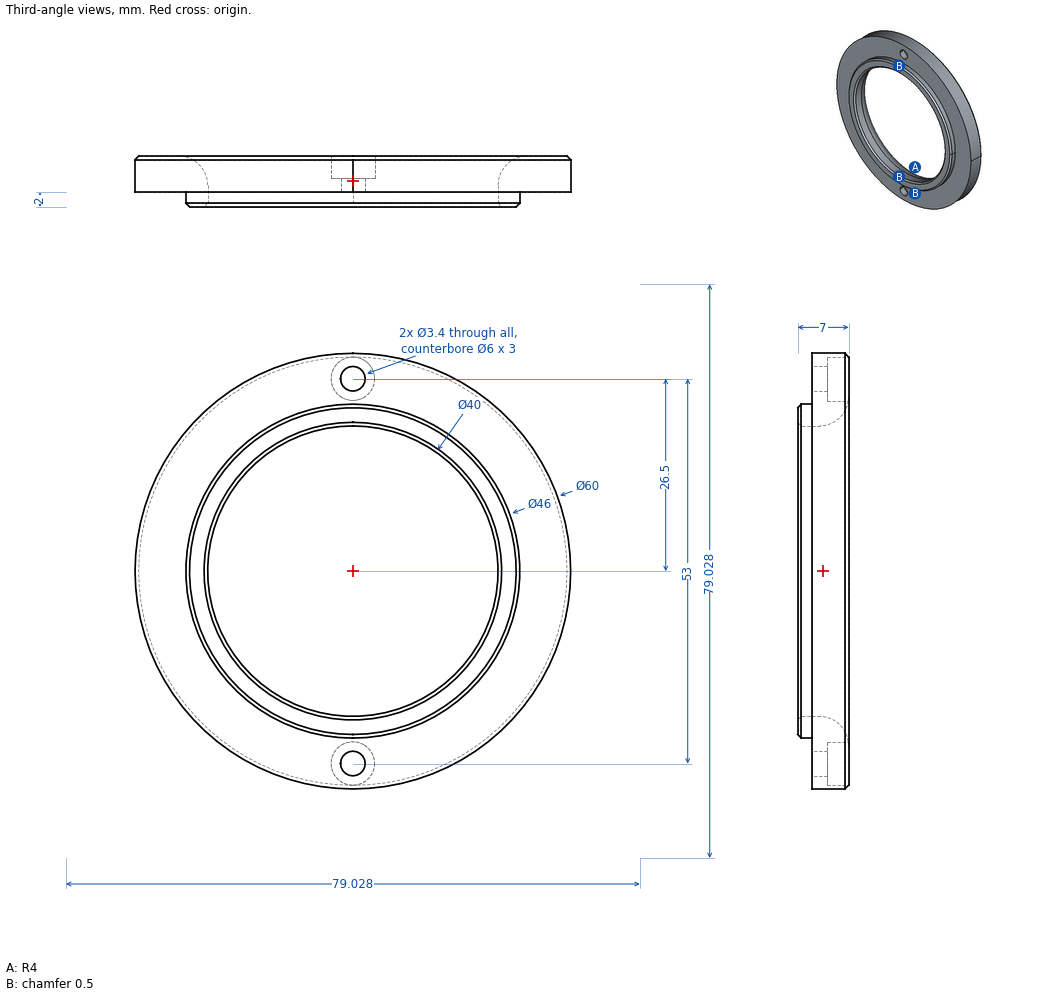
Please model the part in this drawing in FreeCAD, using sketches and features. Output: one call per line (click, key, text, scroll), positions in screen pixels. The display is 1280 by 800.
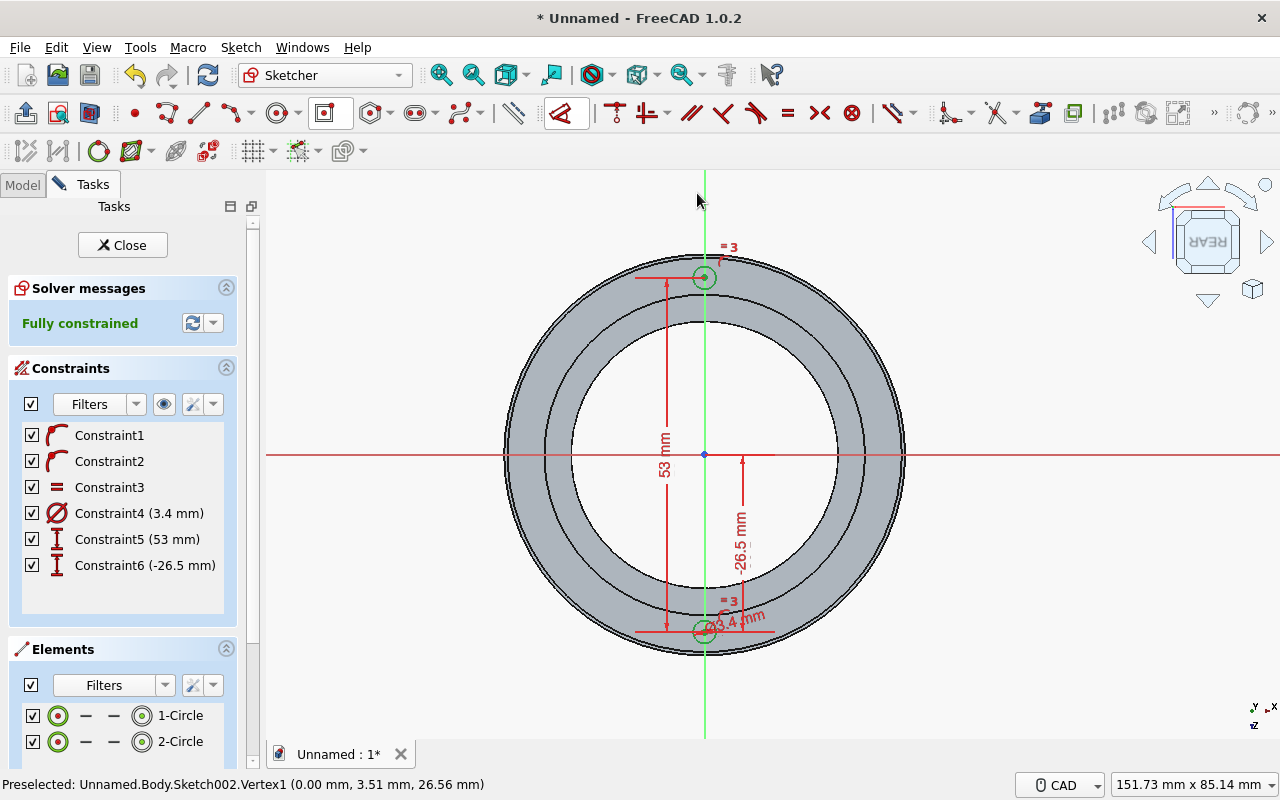
click(123, 245)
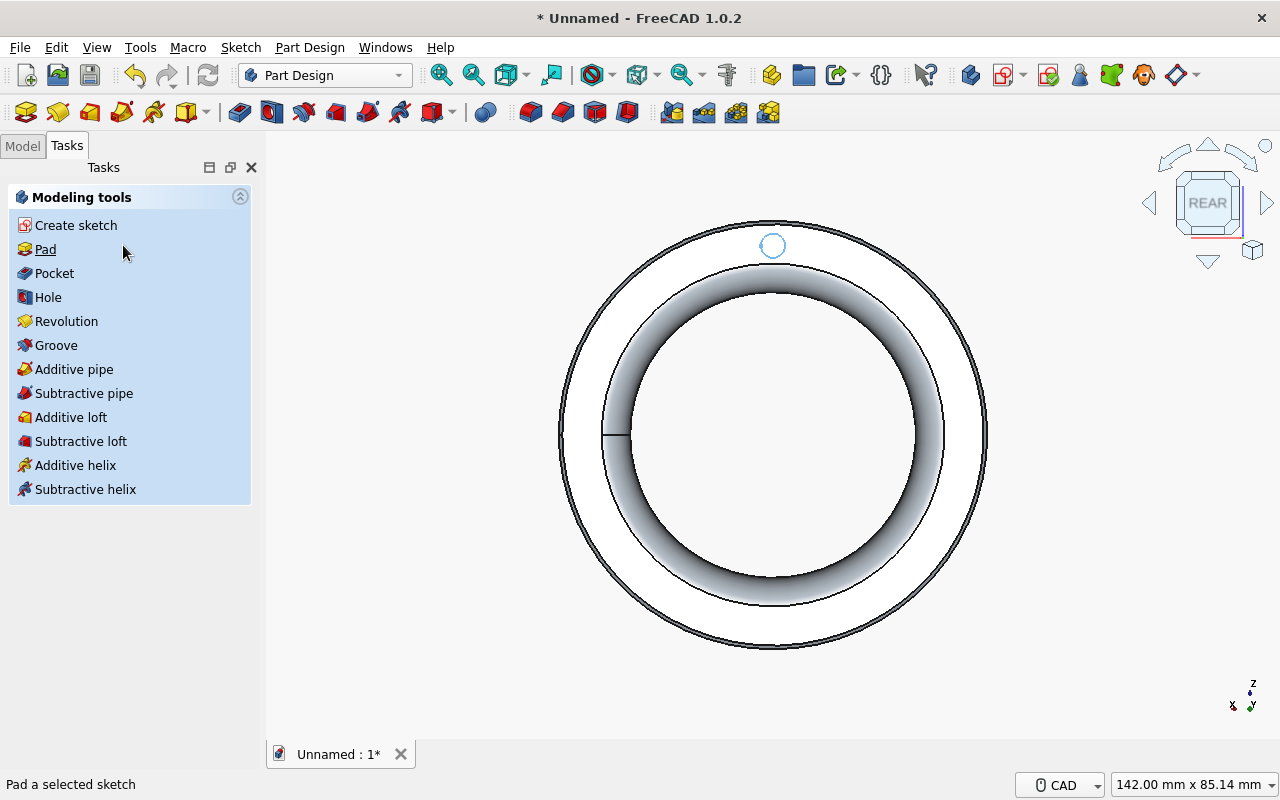
click(272, 112)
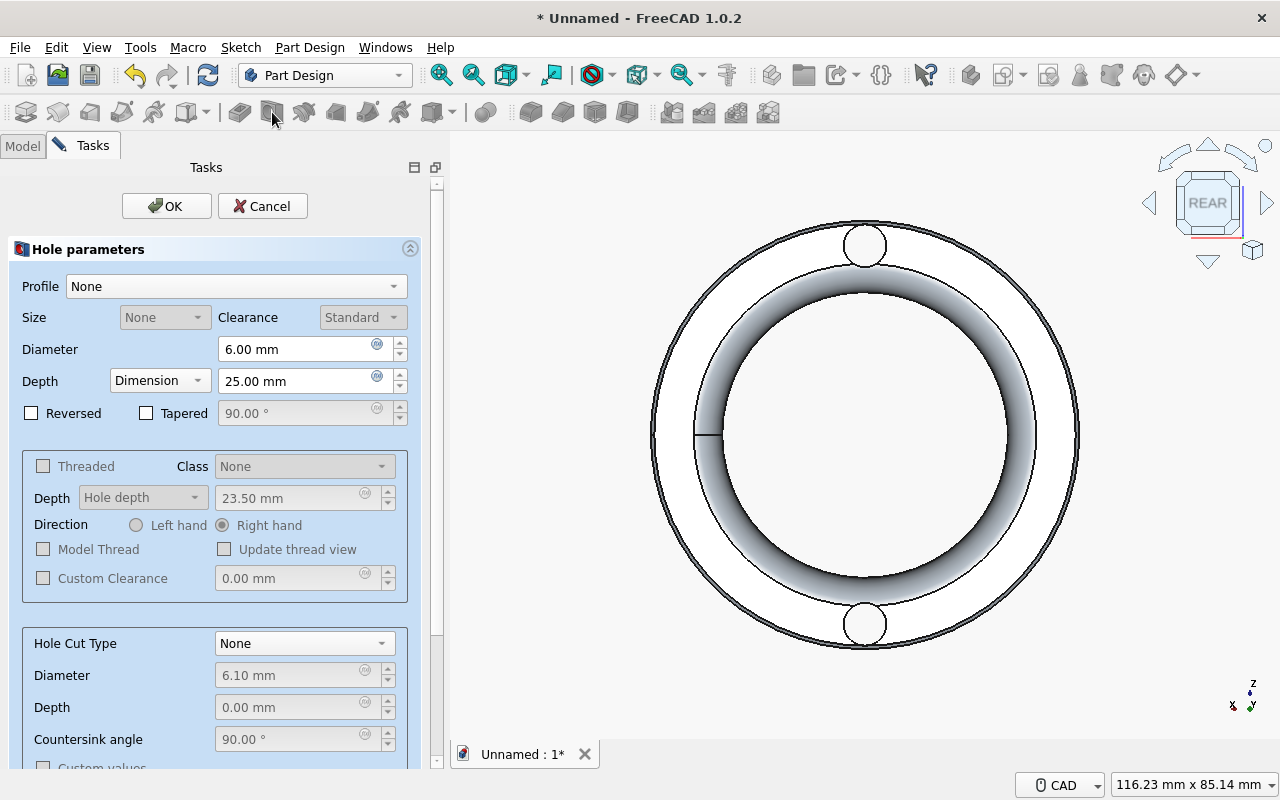
triple_click(305, 349)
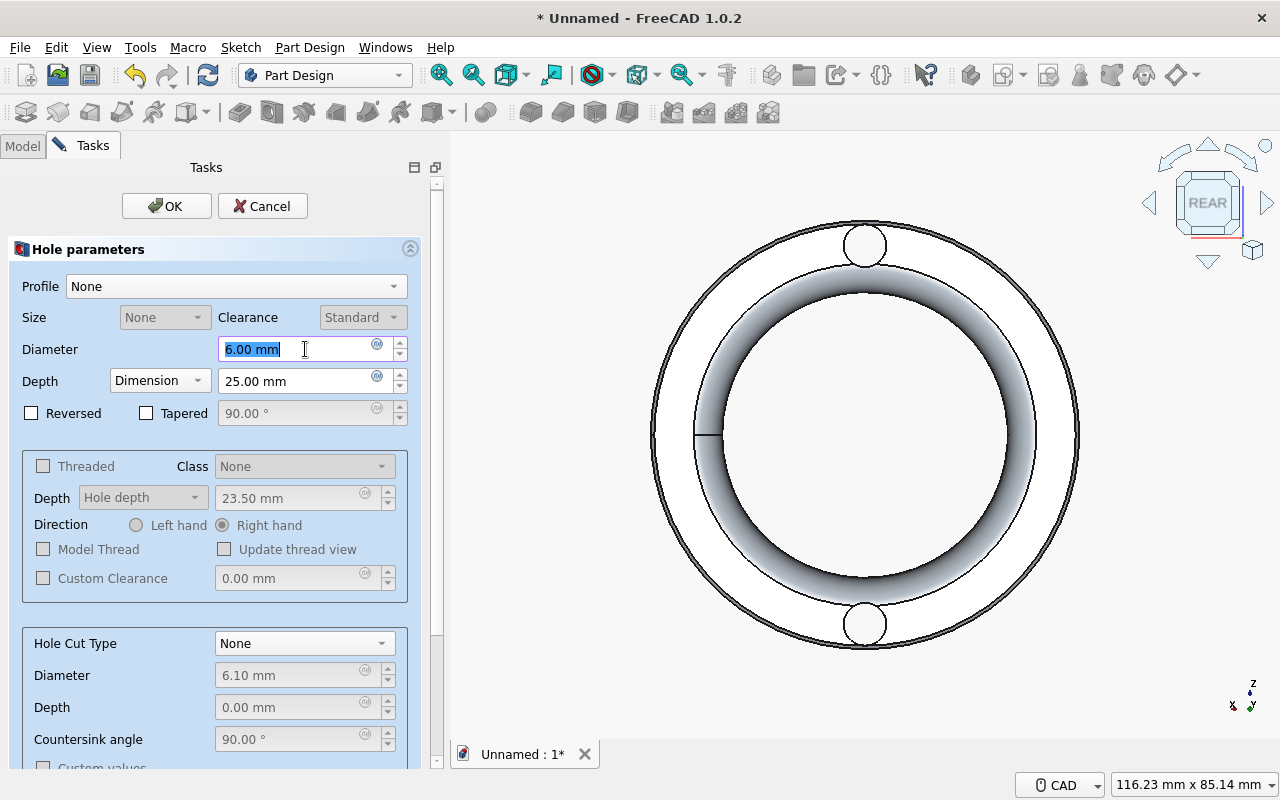
text(3.4)
key(Tab)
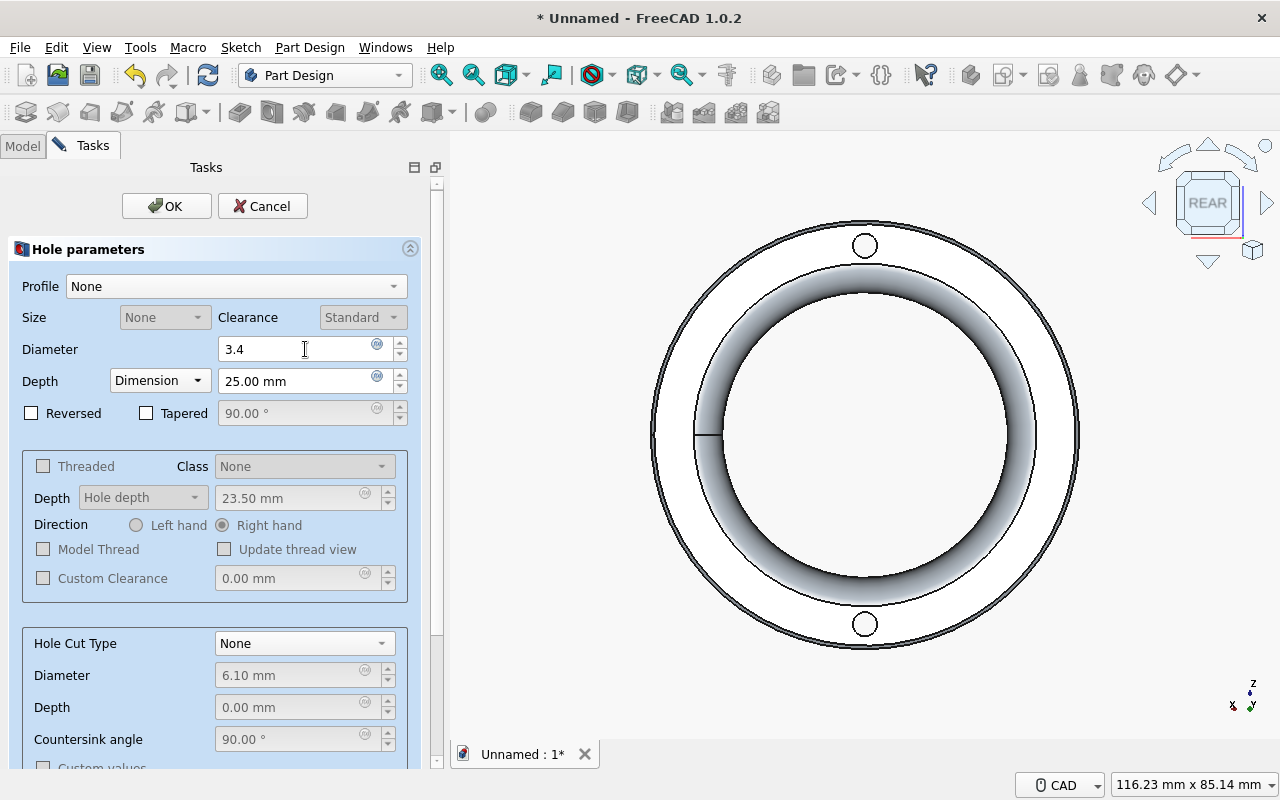
click(161, 380)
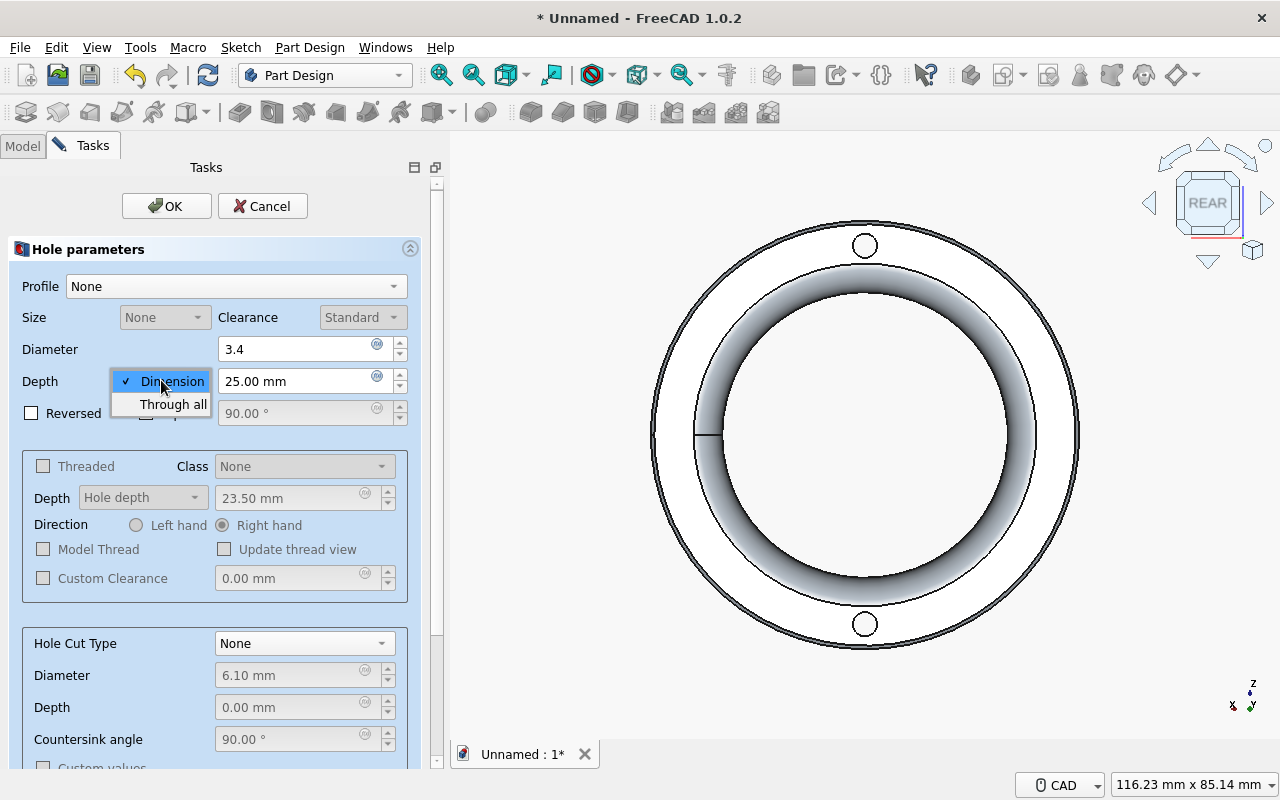
click(160, 404)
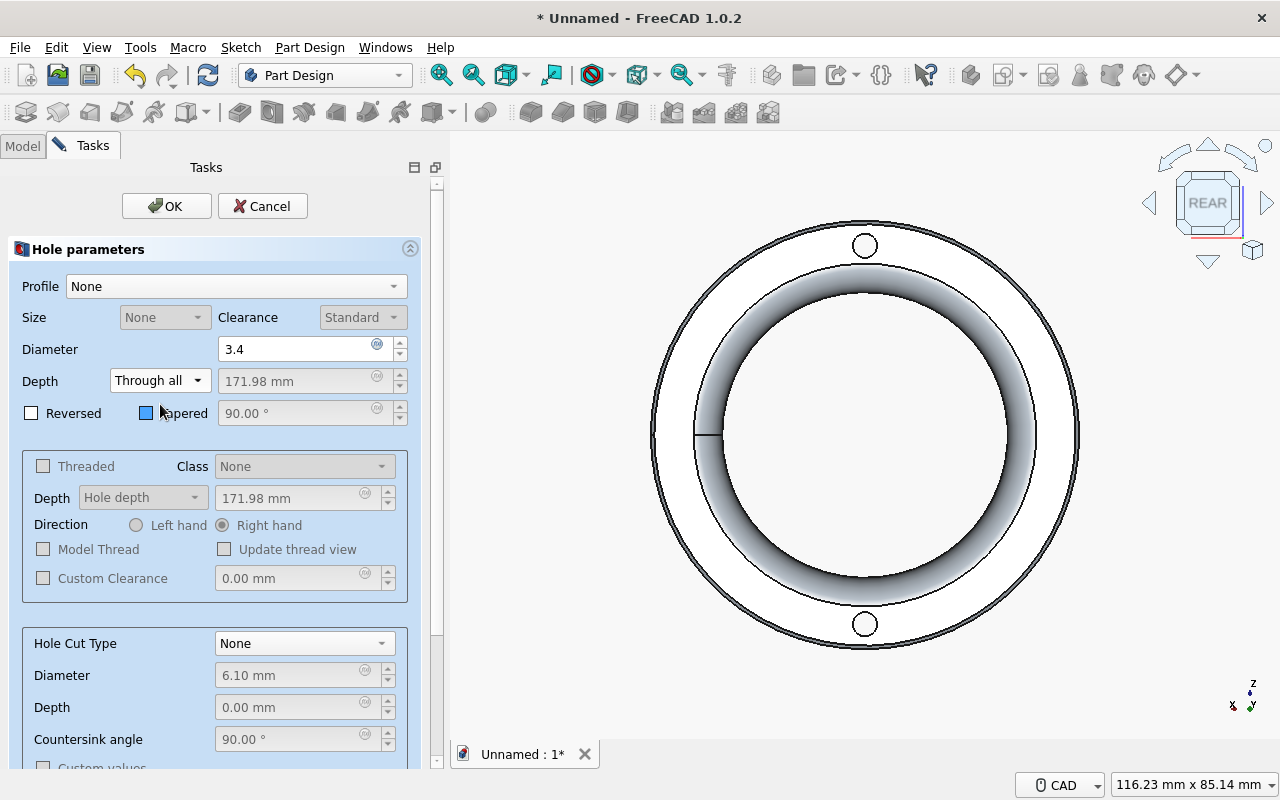
click(306, 644)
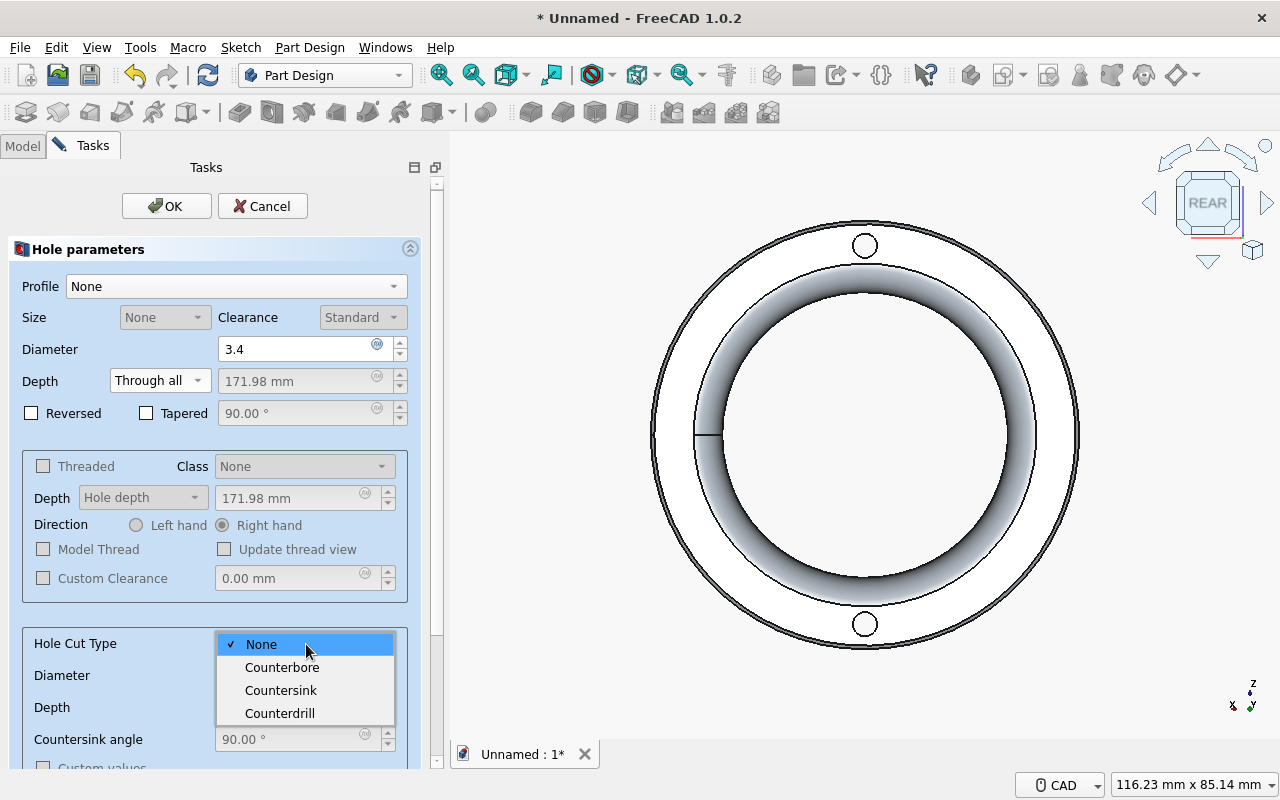
click(304, 668)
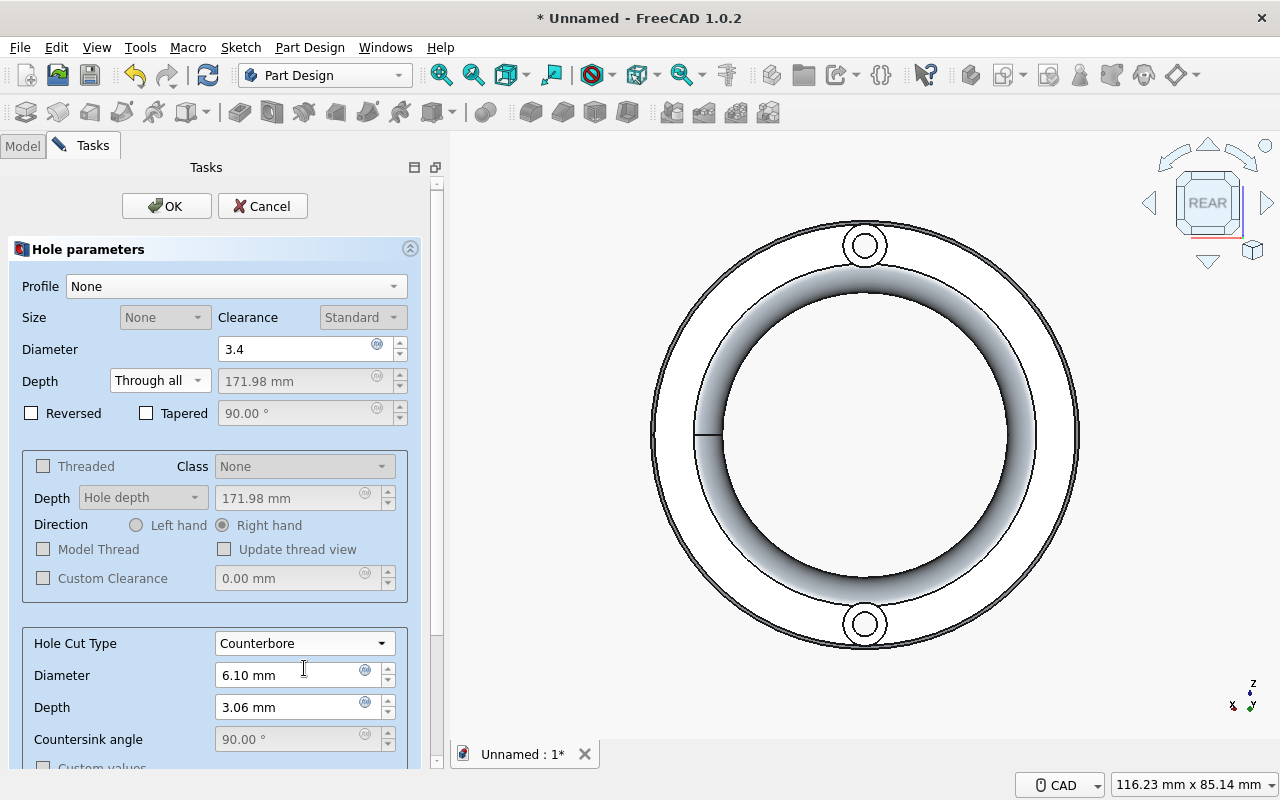
triple_click(298, 675)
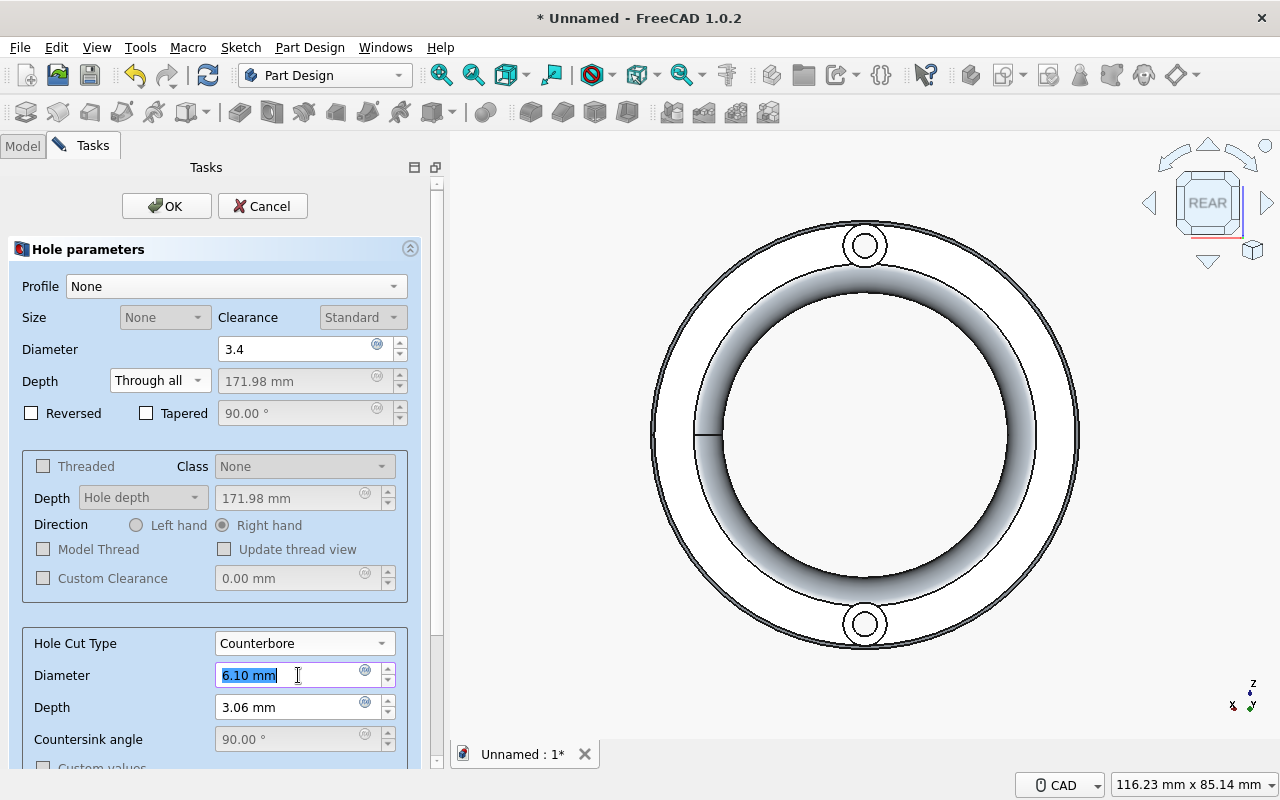
text(6)
key(Tab)